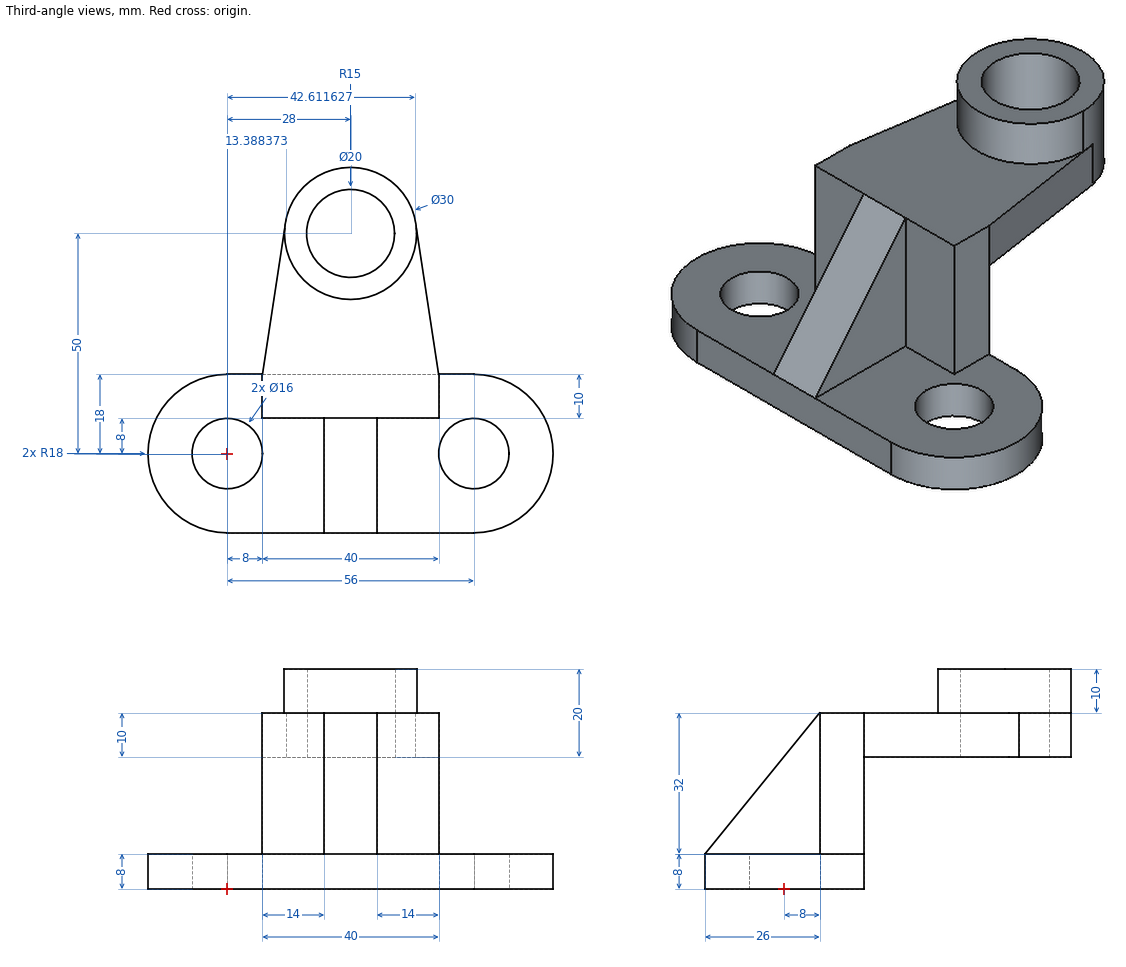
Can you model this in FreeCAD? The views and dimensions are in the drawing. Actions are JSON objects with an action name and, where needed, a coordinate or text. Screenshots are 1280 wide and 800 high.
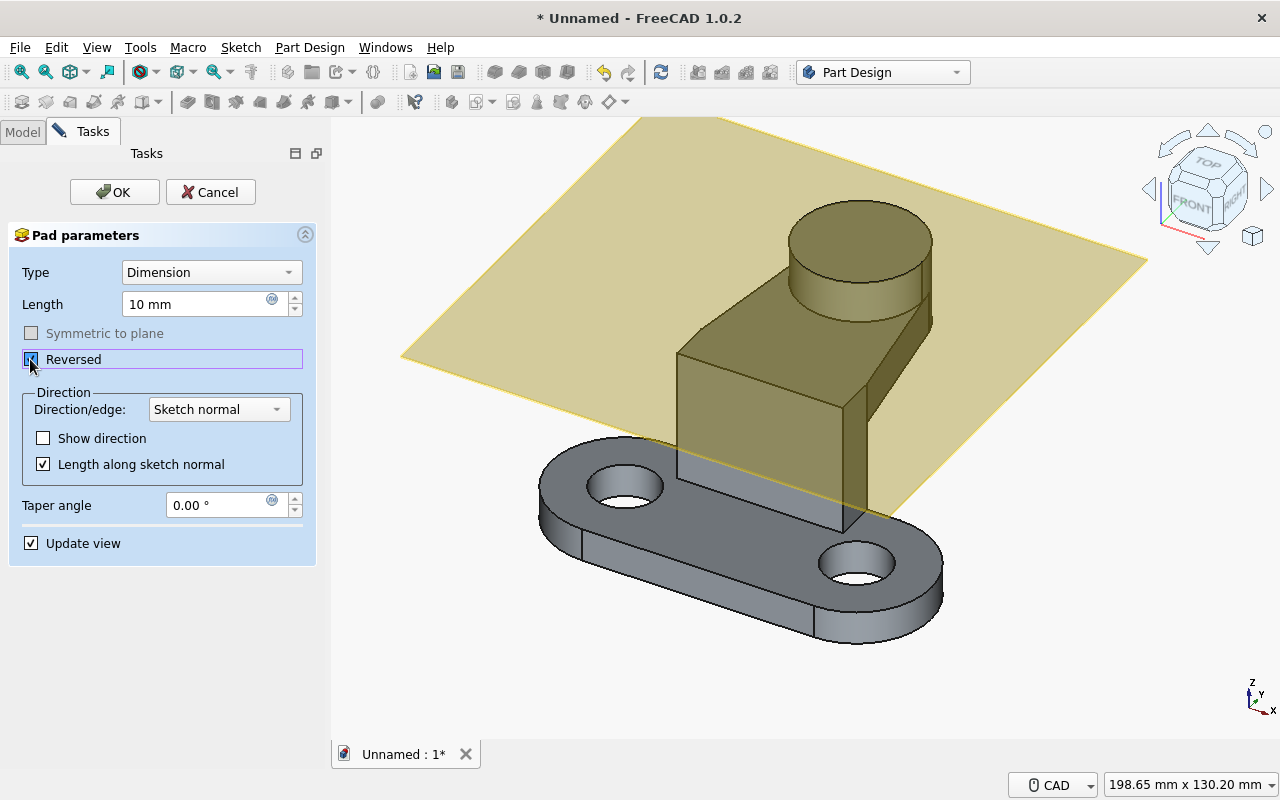
{"action": "left_click", "coordinate": [115, 192]}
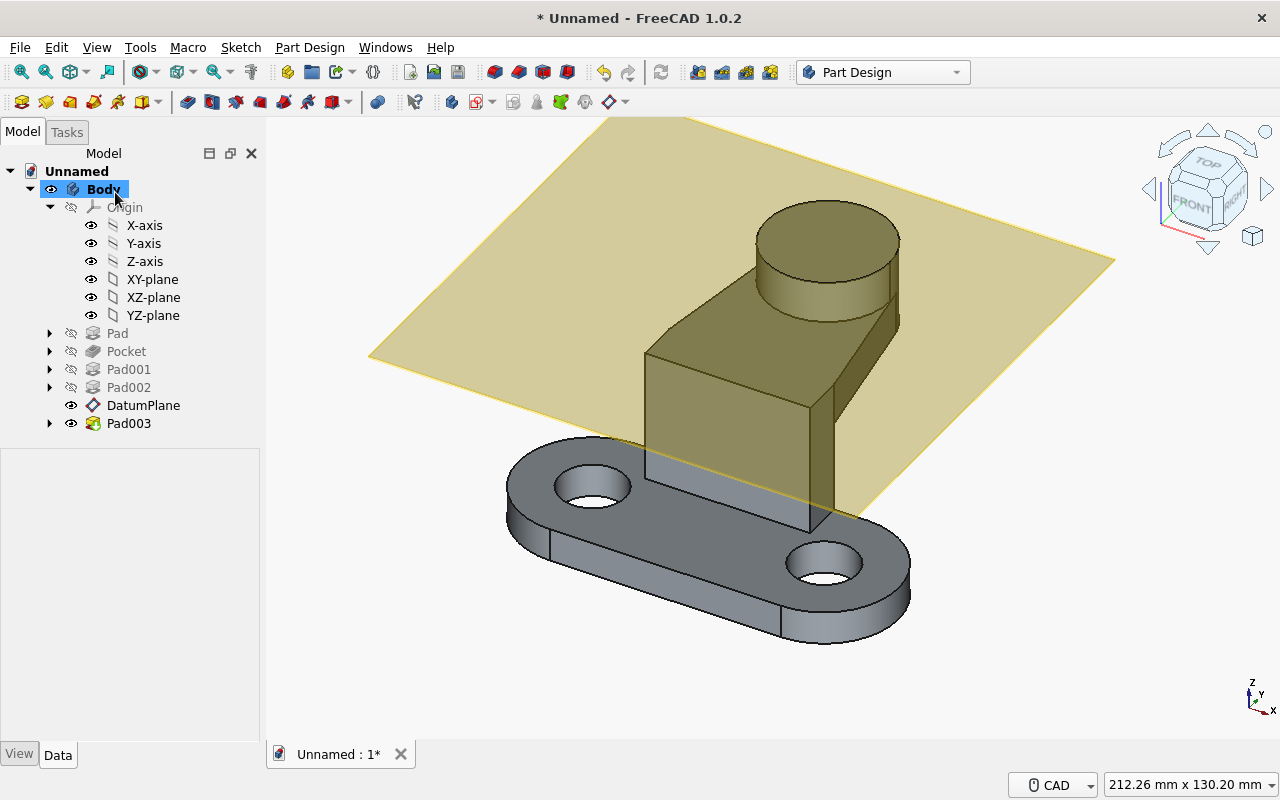
{"action": "left_click", "coordinate": [116, 405]}
{"action": "key", "text": "space"}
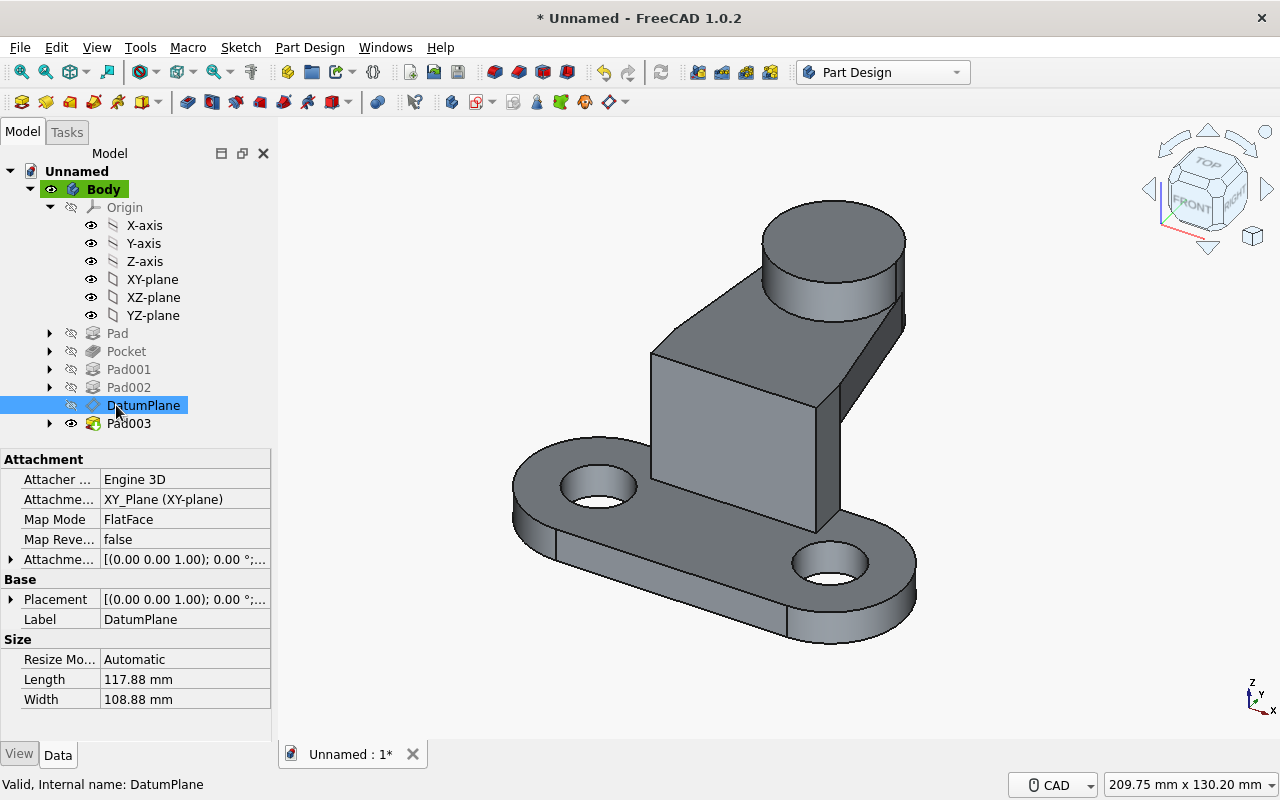
{"action": "left_click", "coordinate": [834, 241]}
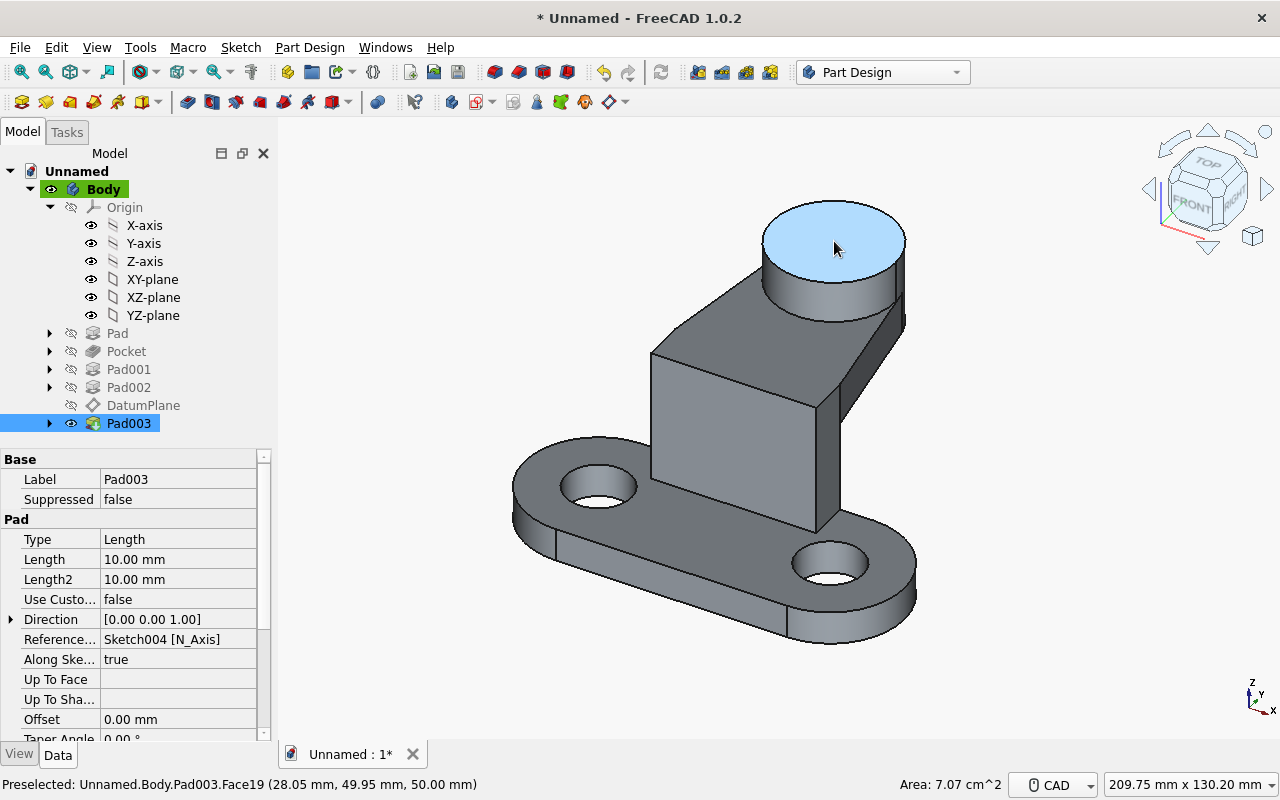
{"action": "left_click", "coordinate": [476, 102]}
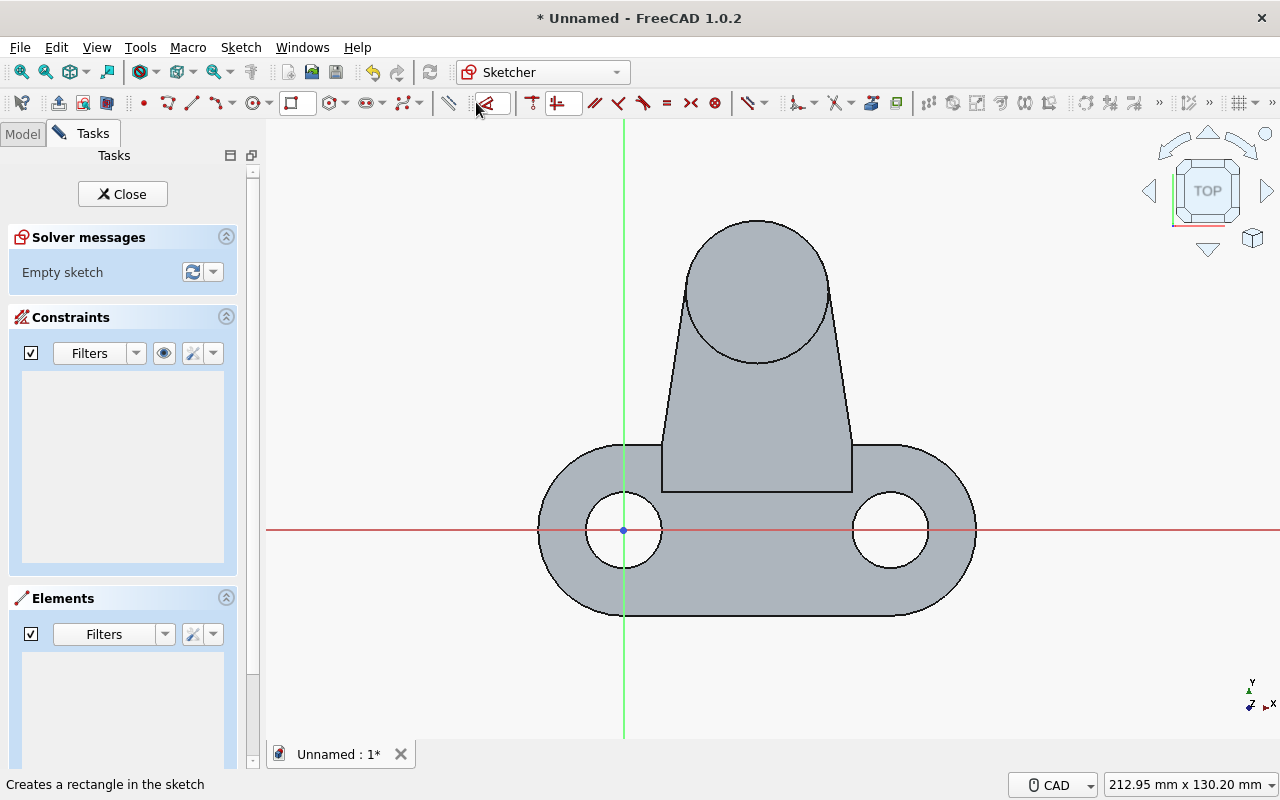
{"action": "scroll", "coordinate": [774, 247], "scroll_direction": "up", "scroll_amount": 7}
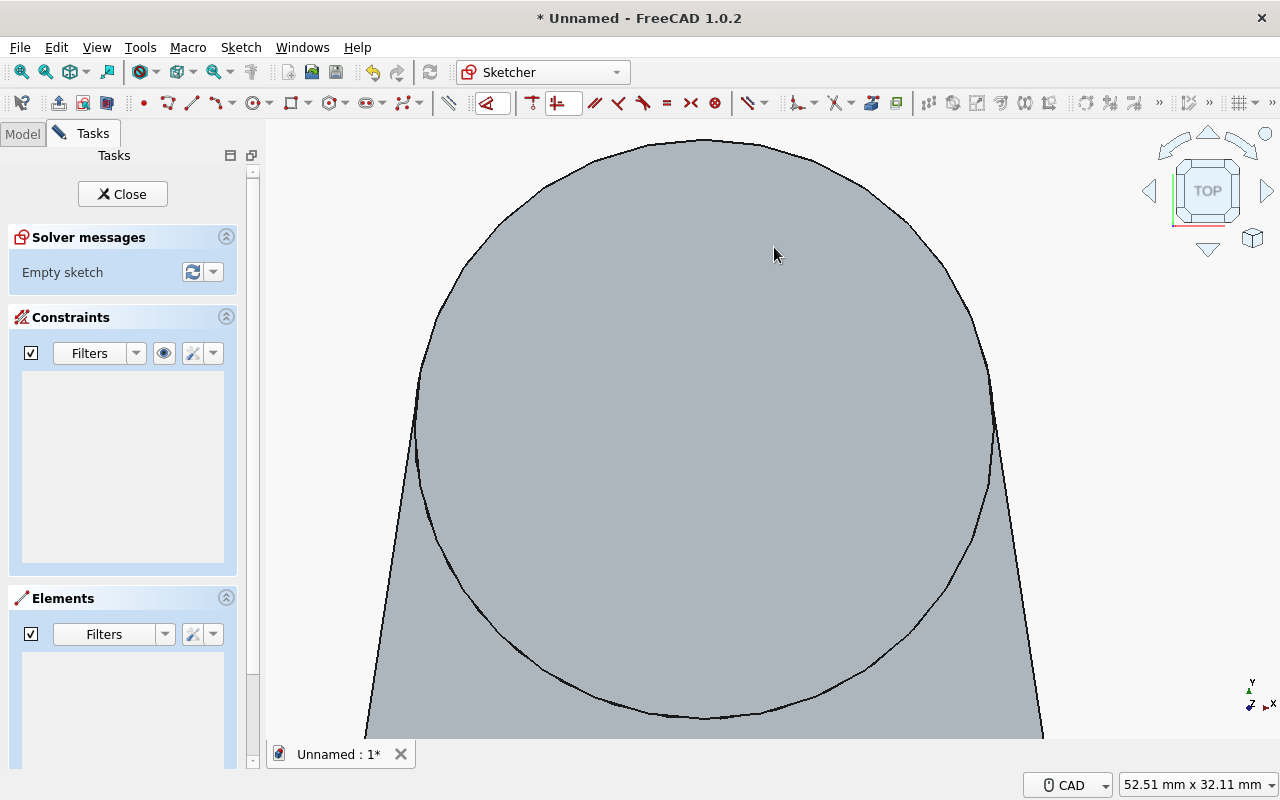
{"action": "left_click", "coordinate": [254, 104]}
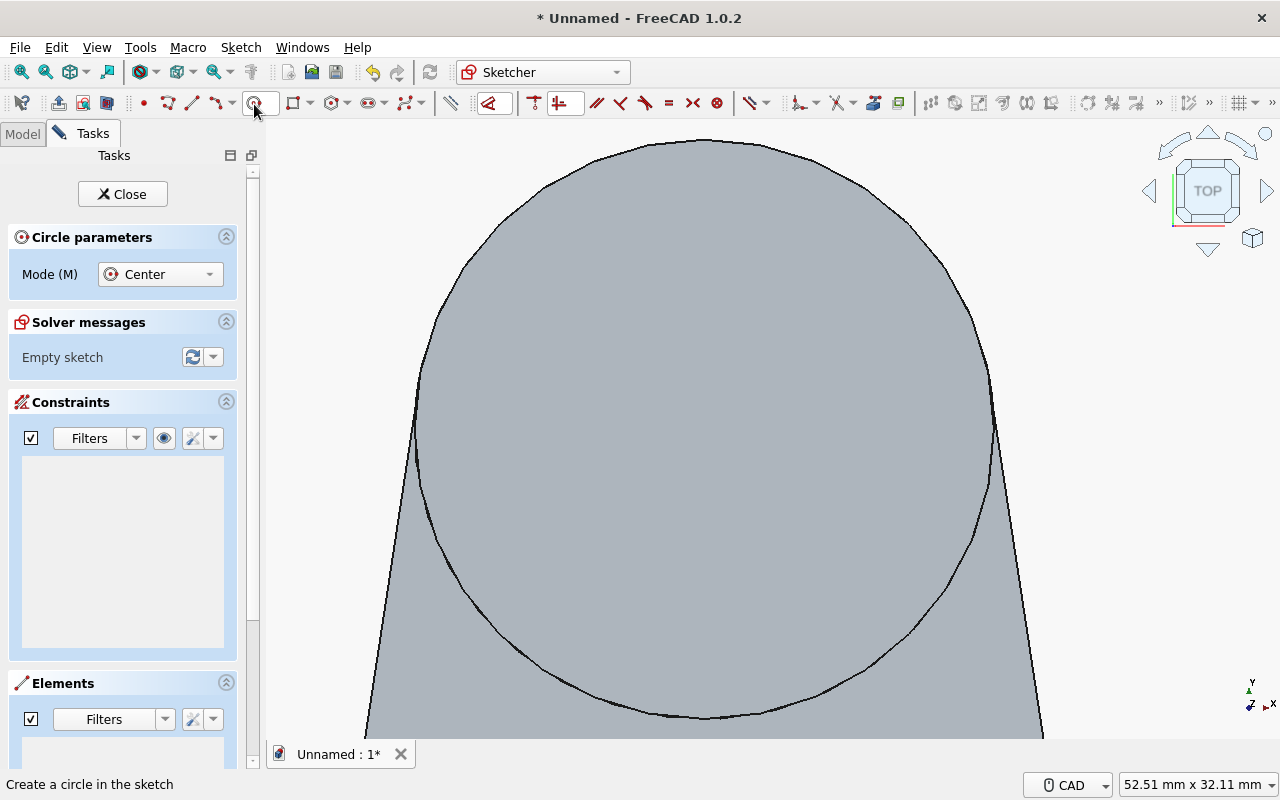
{"action": "left_click", "coordinate": [704, 429]}
{"action": "mouse_move", "coordinate": [841, 293]}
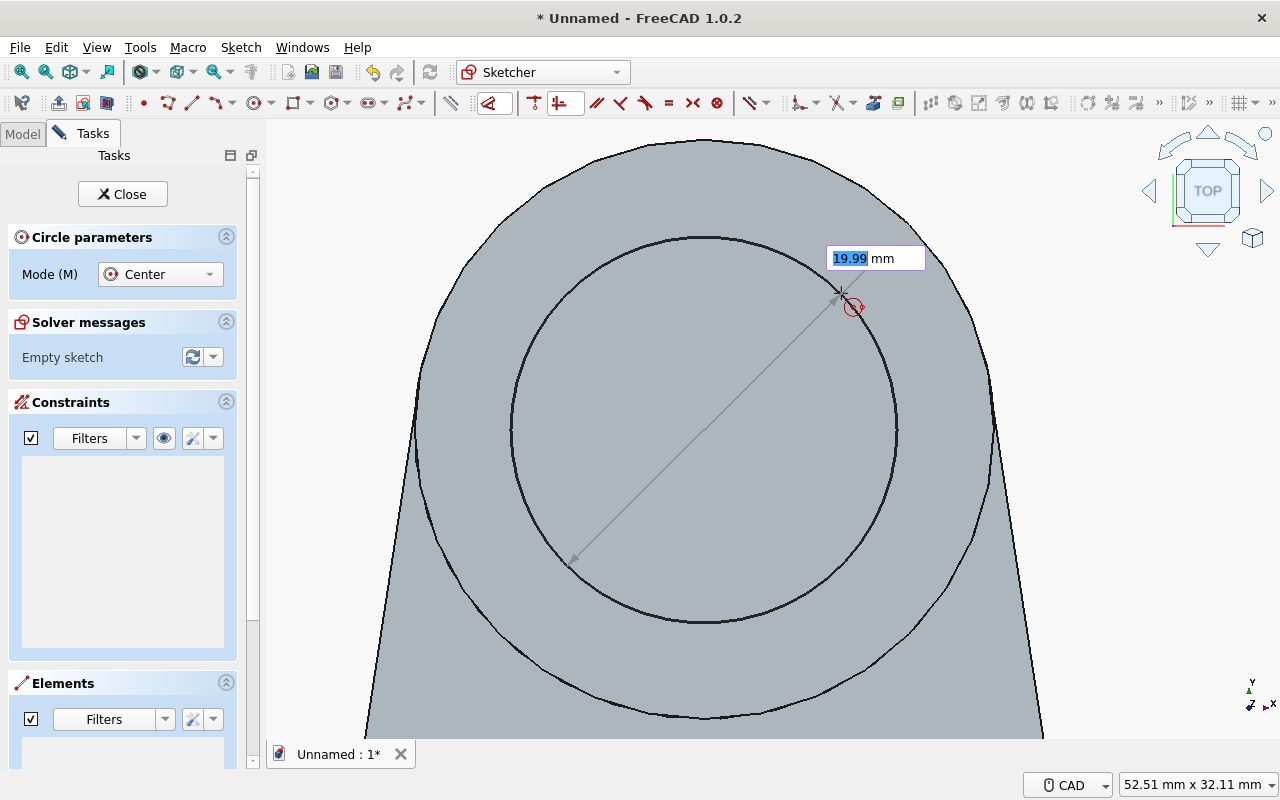
{"action": "type", "text": "20"}
{"action": "key", "text": "Return"}
{"action": "key", "text": "Escape"}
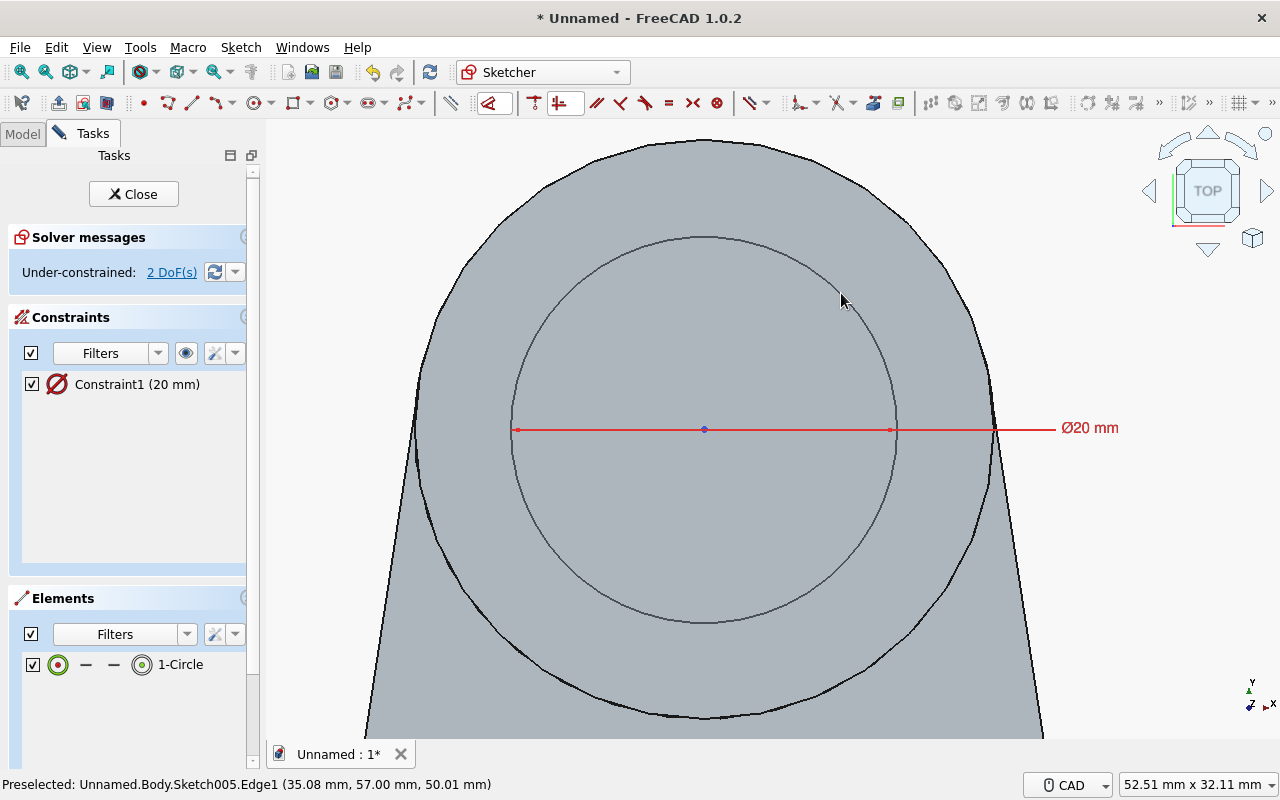
{"action": "left_click", "coordinate": [704, 430]}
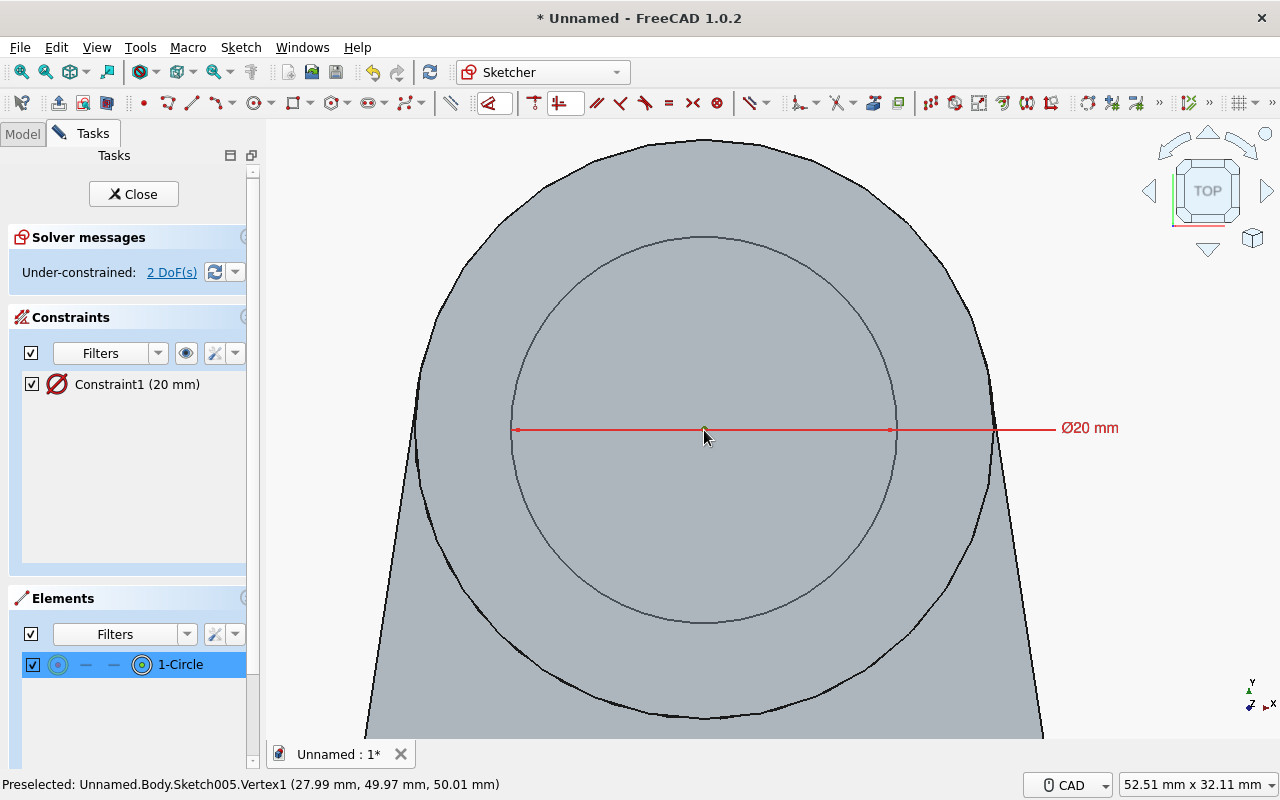
{"action": "key", "text": "l"}